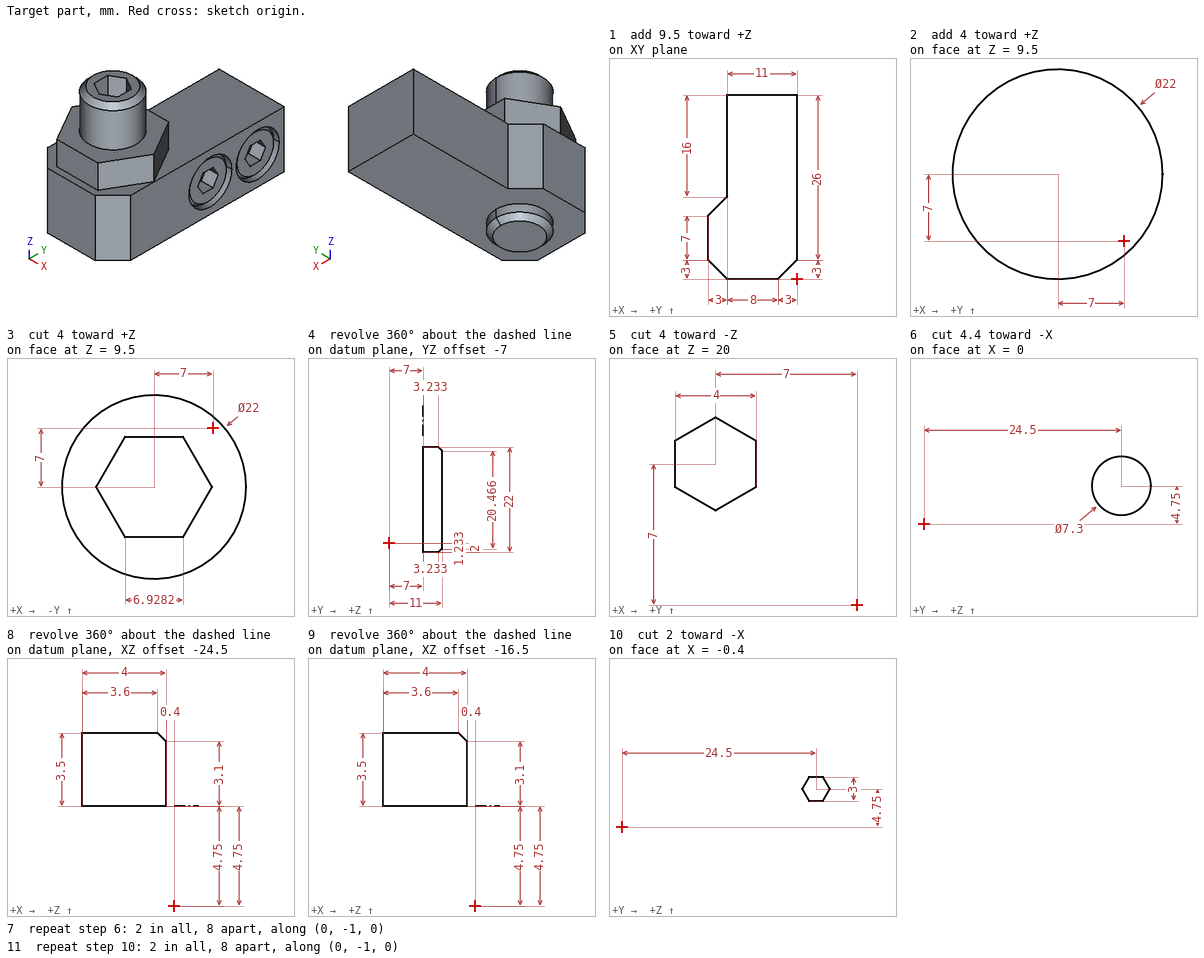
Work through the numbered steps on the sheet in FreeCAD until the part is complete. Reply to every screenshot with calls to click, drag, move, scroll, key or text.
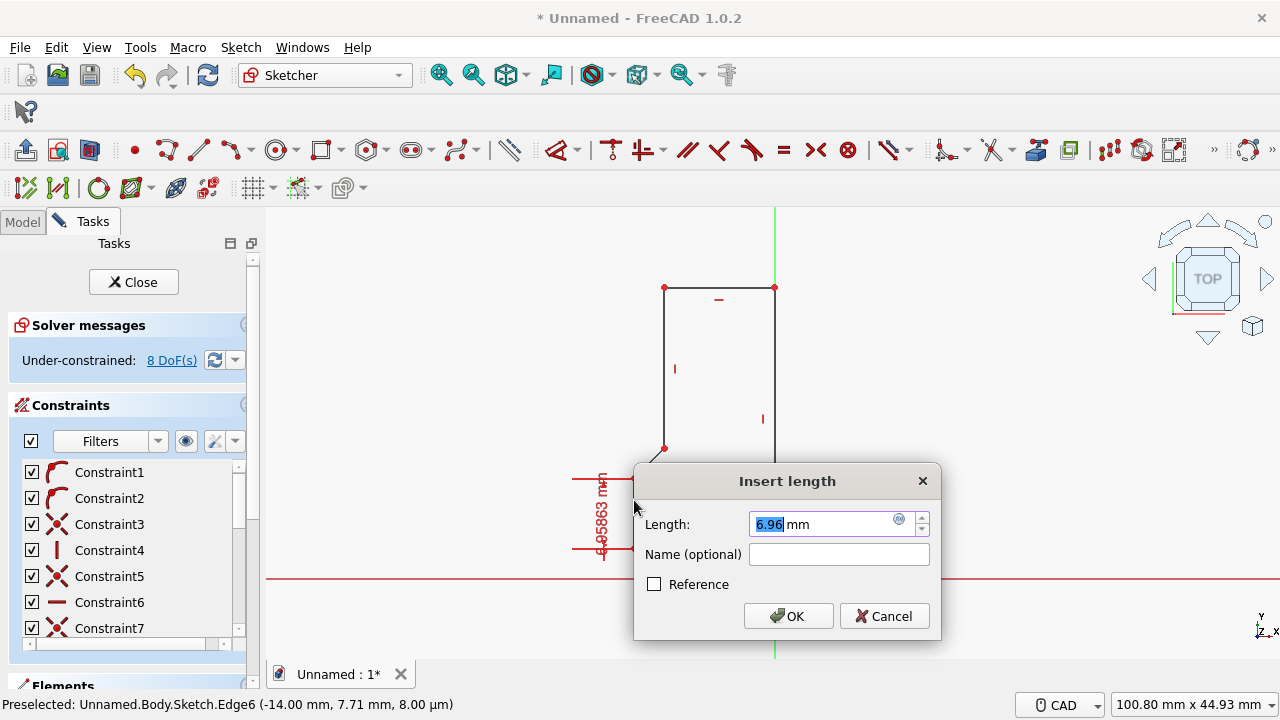
text(7)
key(Return)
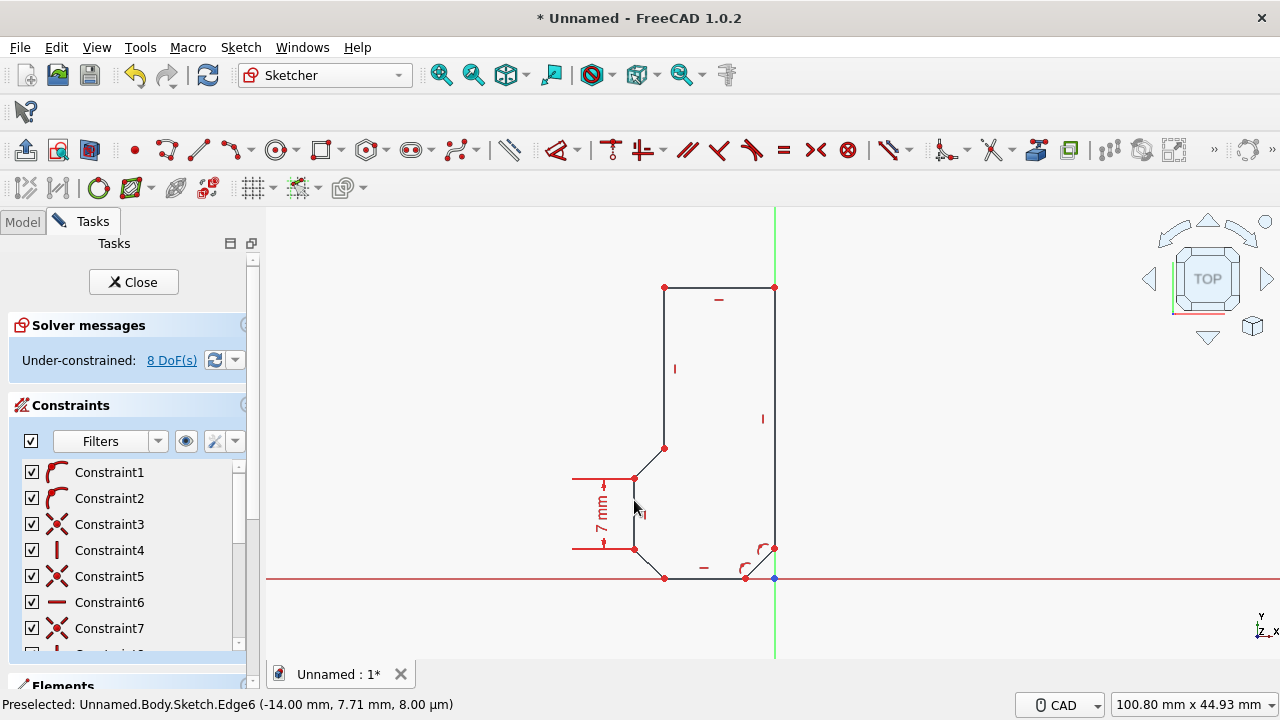
click(688, 579)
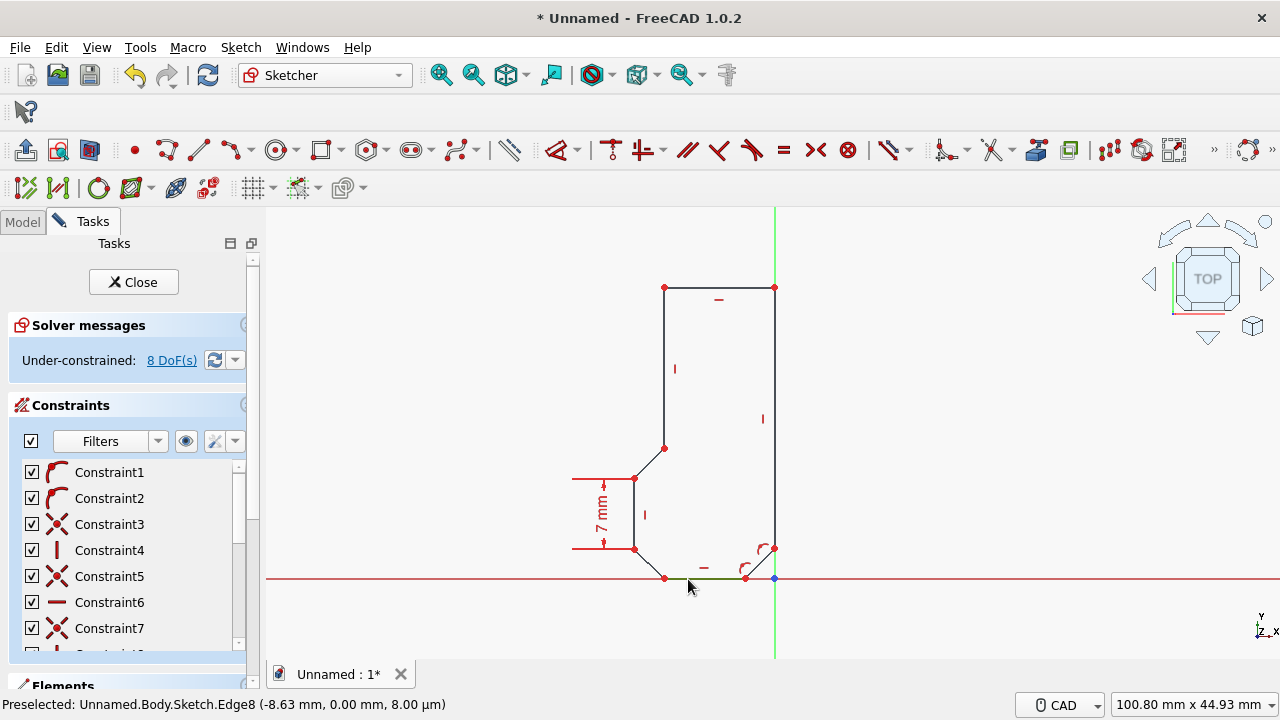
click(580, 150)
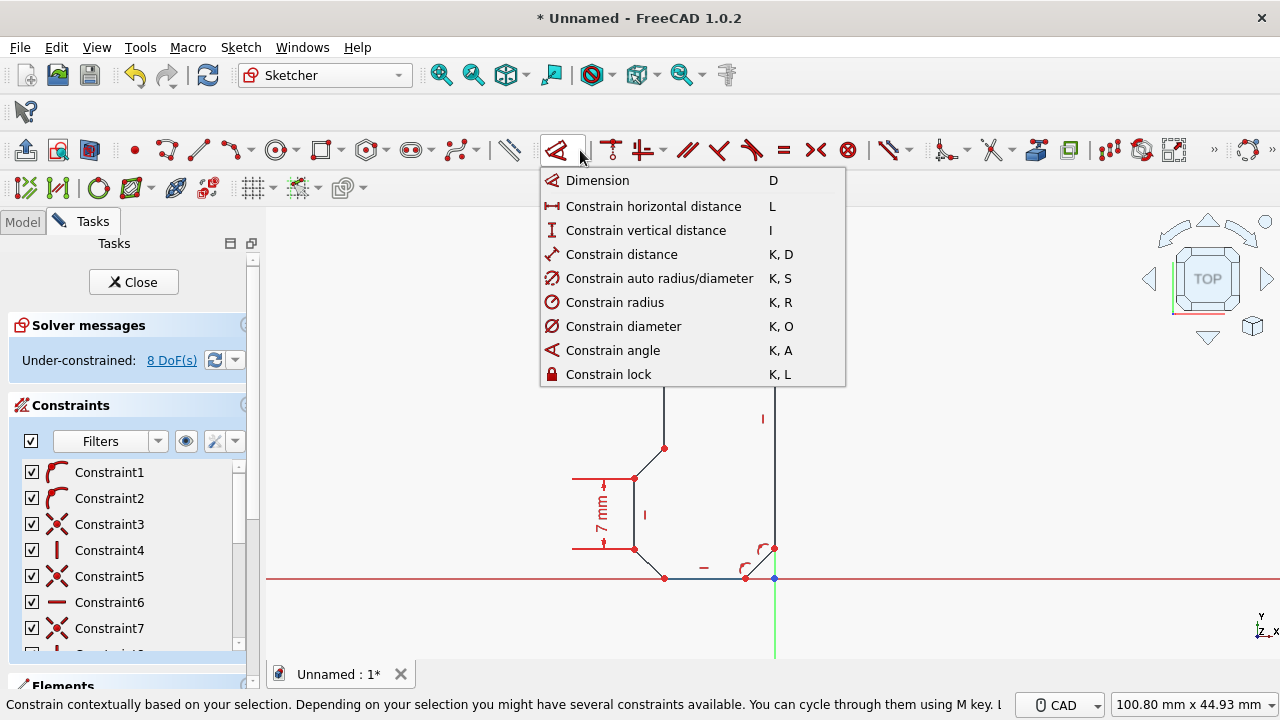
click(693, 206)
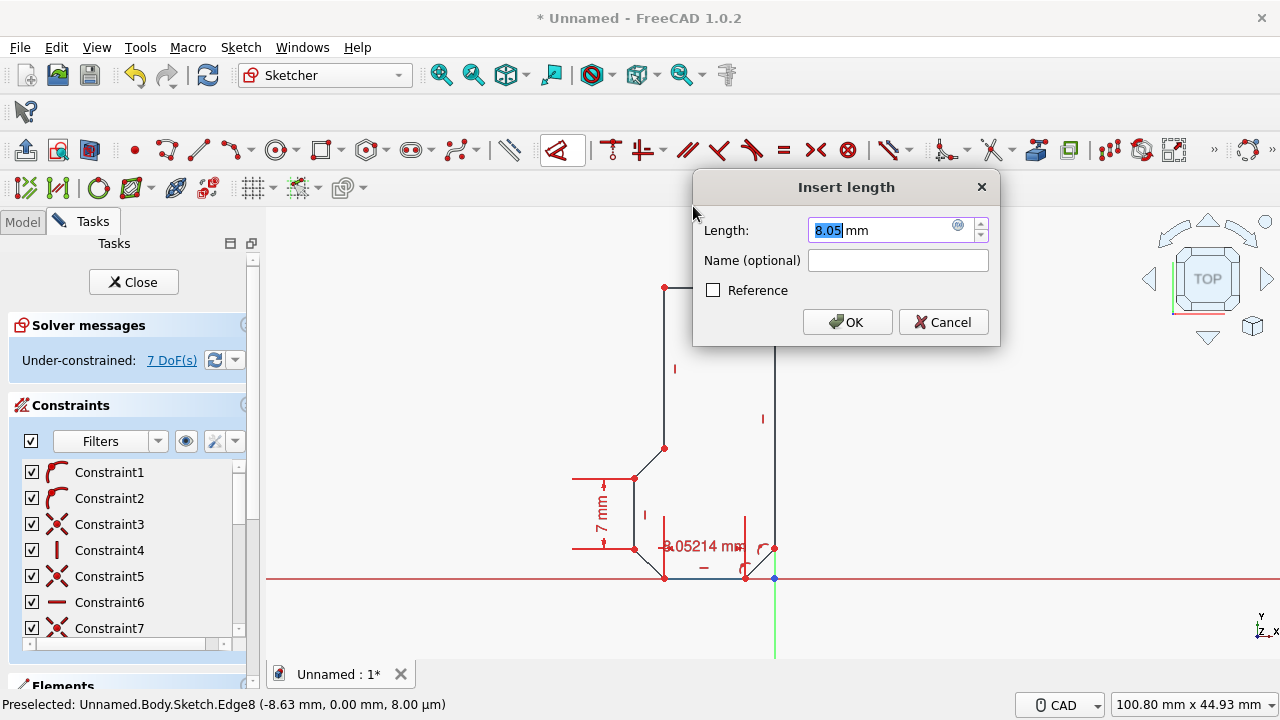
text(8)
key(Return)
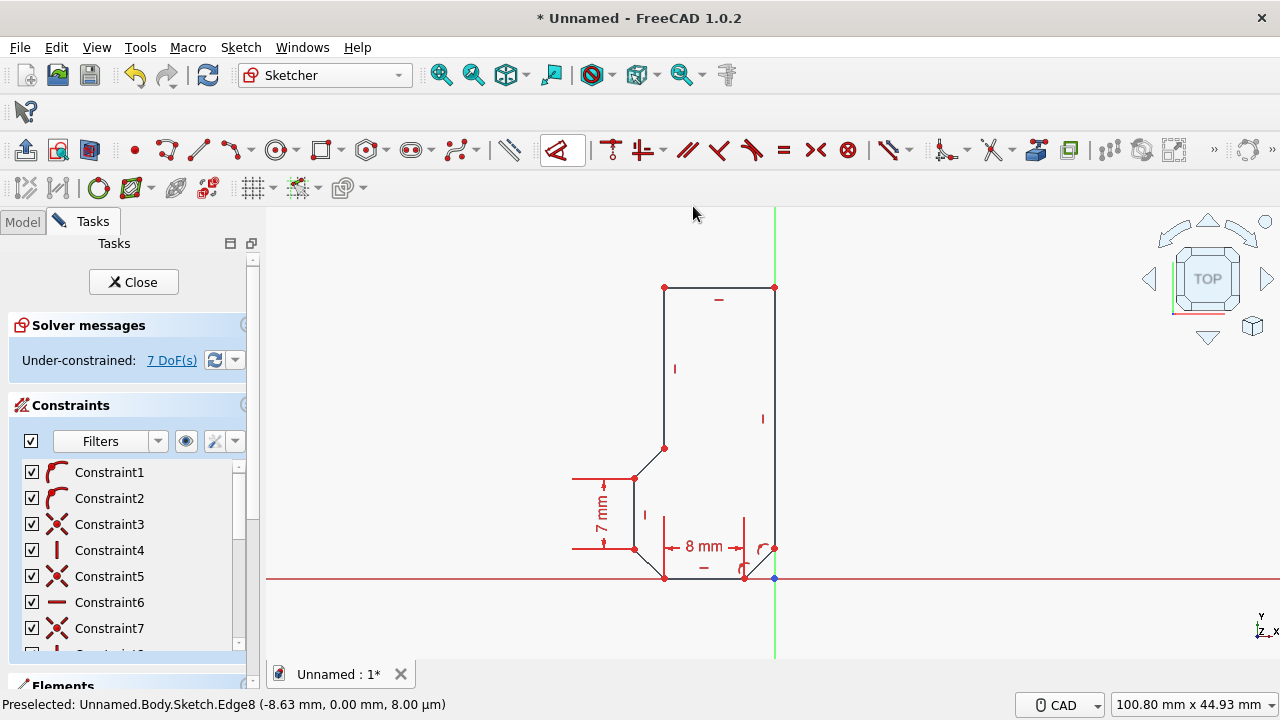
click(775, 471)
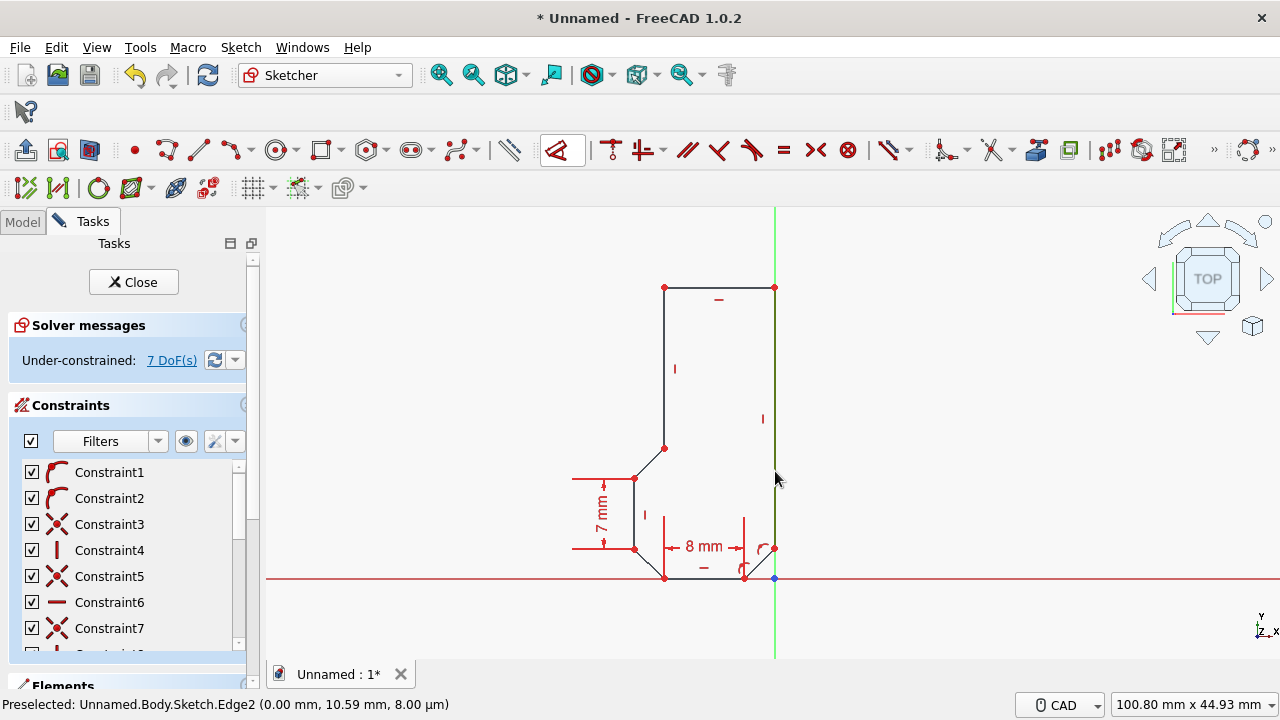
key(i)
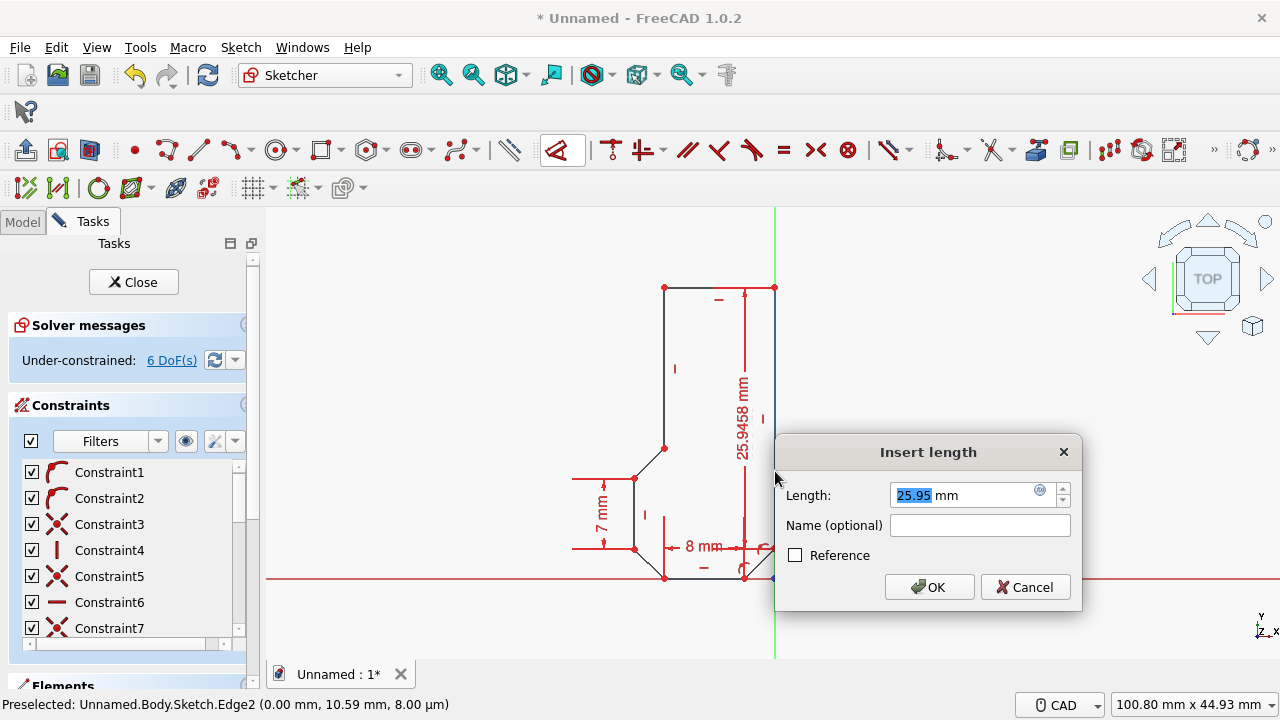
text(26)
key(Return)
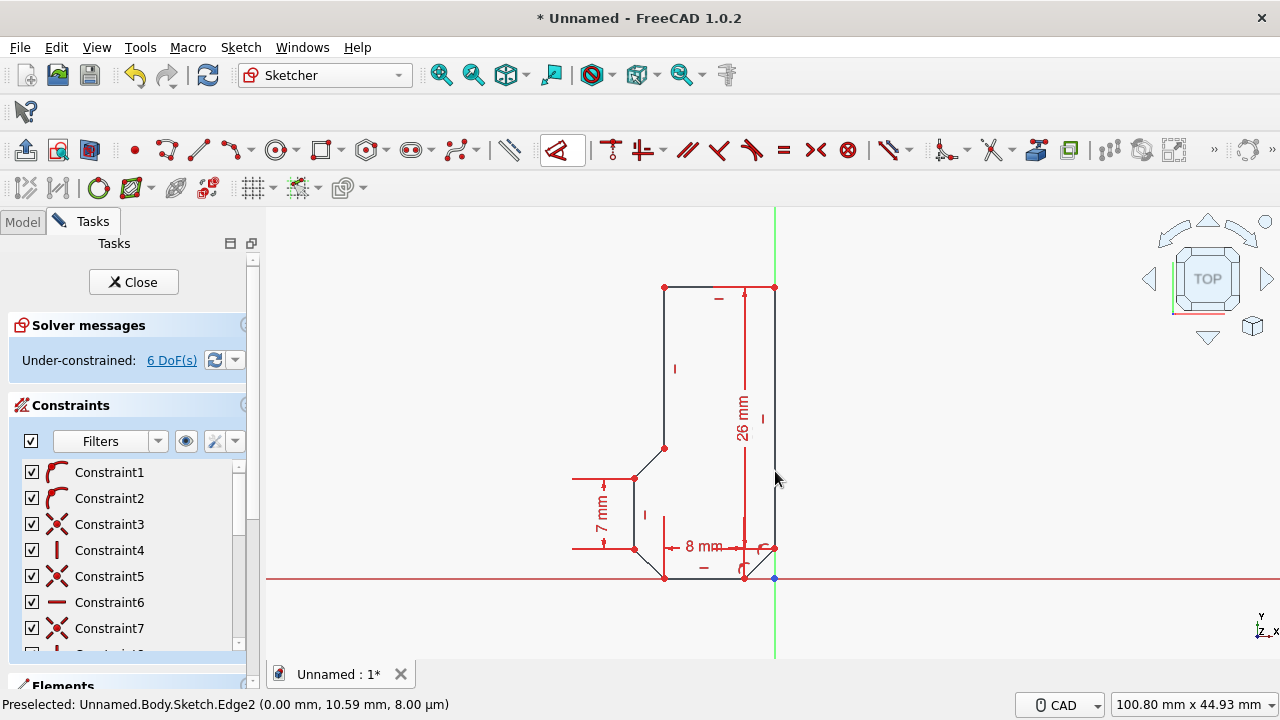
click(742, 287)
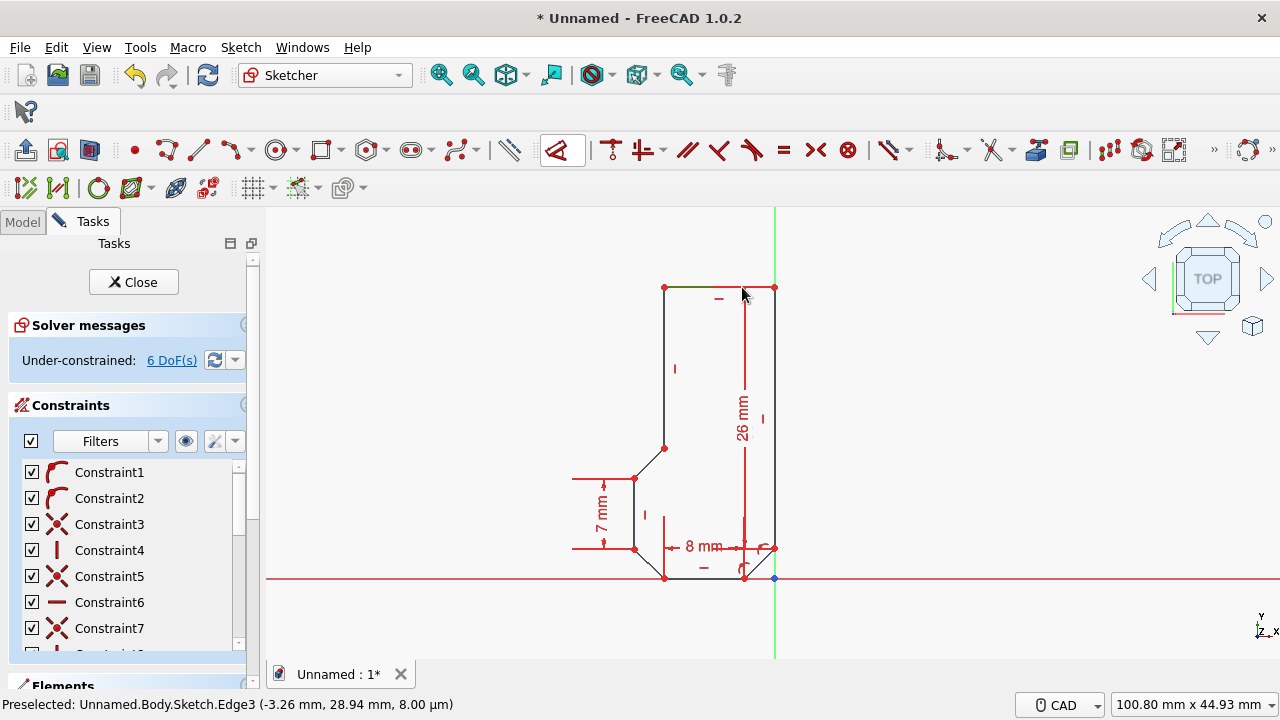
key(l)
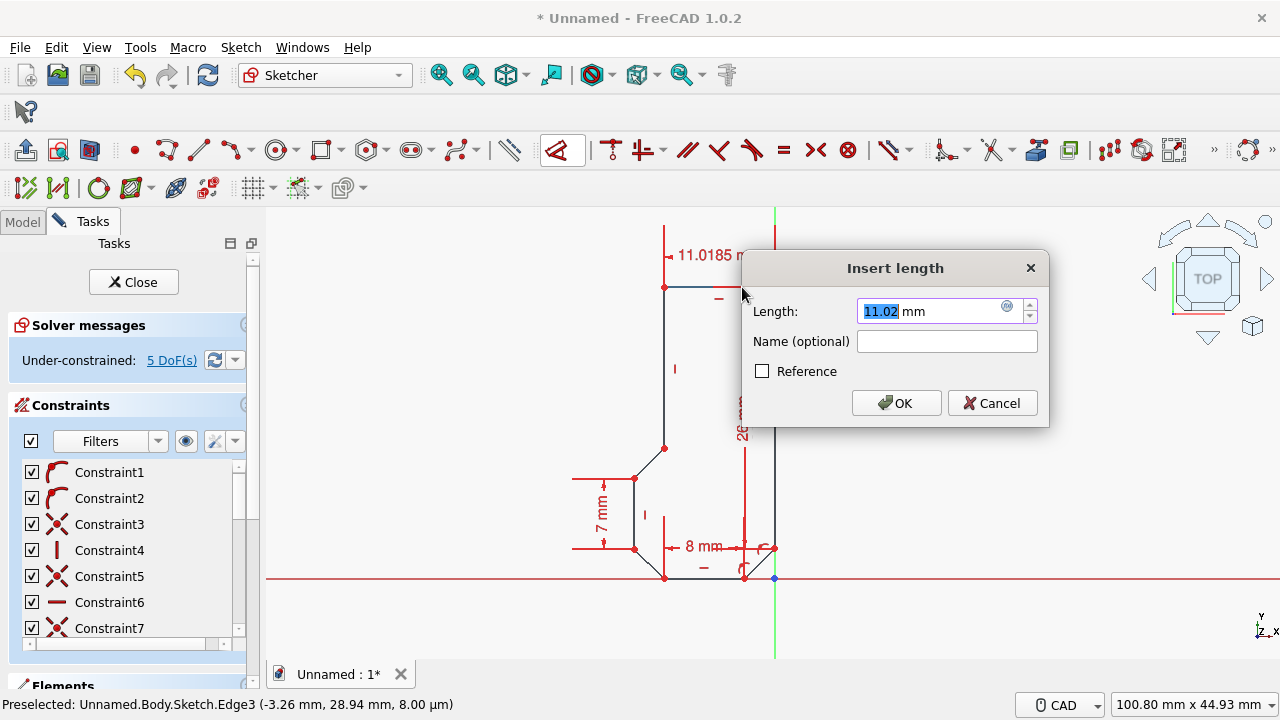
text(11)
key(Return)